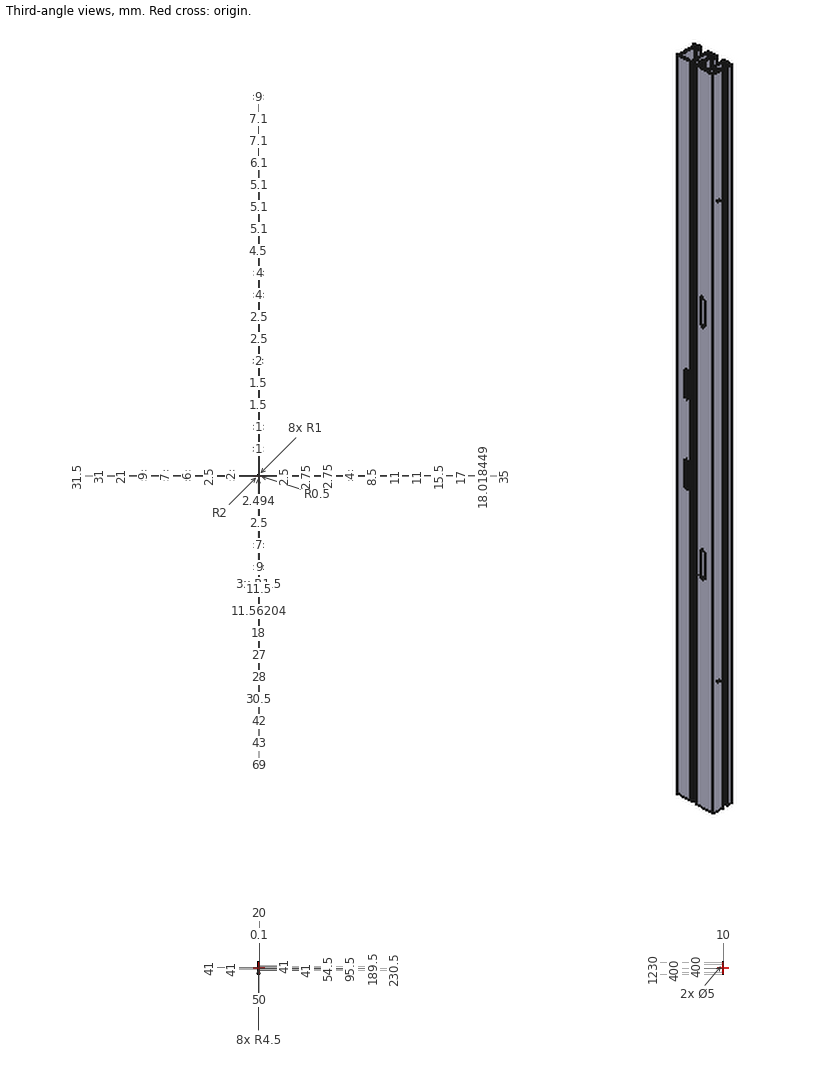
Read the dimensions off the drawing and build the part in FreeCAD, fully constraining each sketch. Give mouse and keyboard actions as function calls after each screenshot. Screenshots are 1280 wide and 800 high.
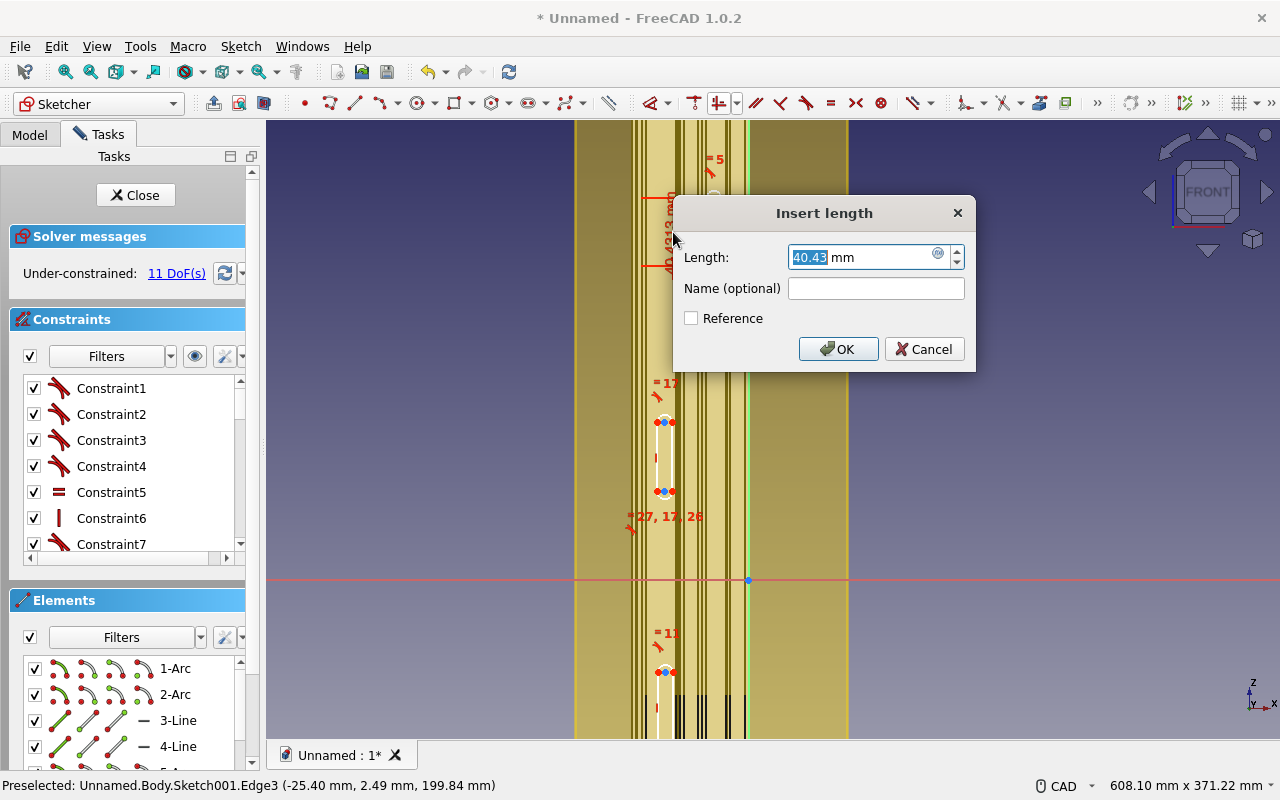
text(41)
key(Return)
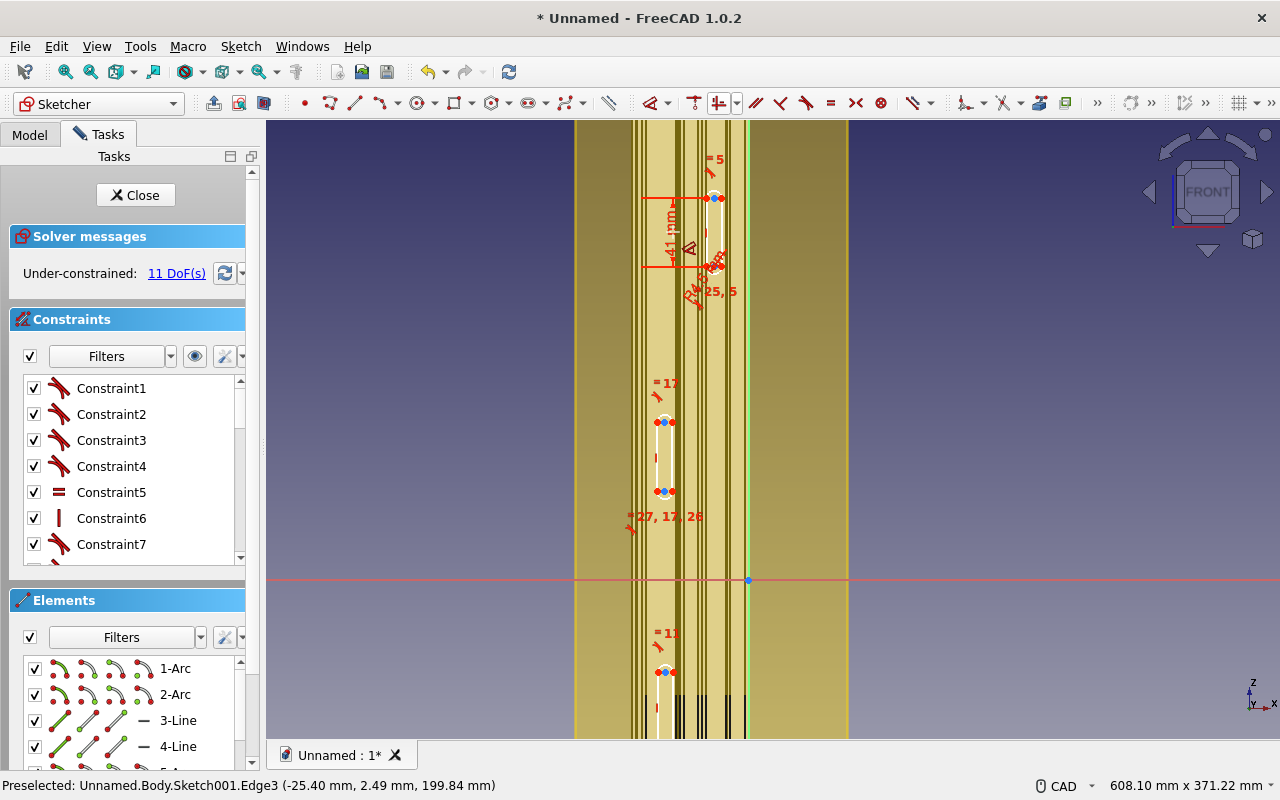
click(658, 693)
click(624, 692)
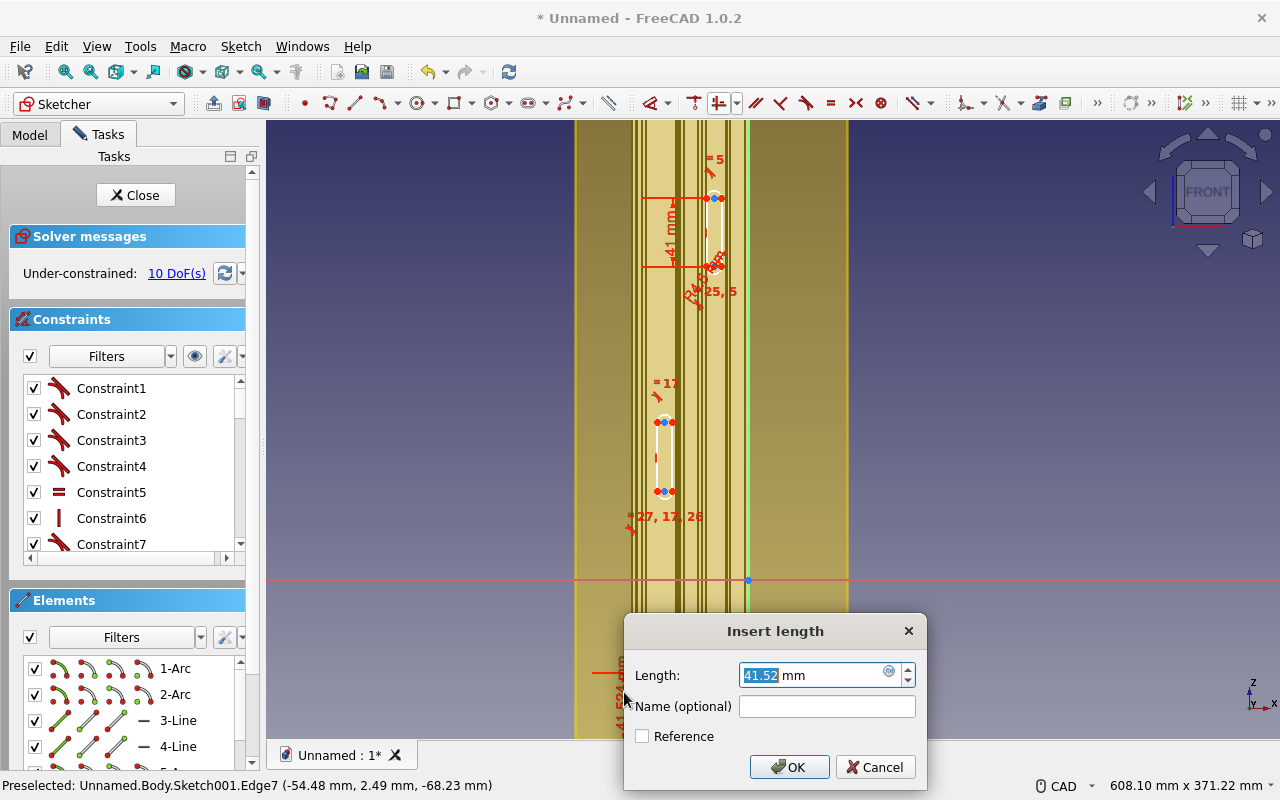
text(41)
key(Return)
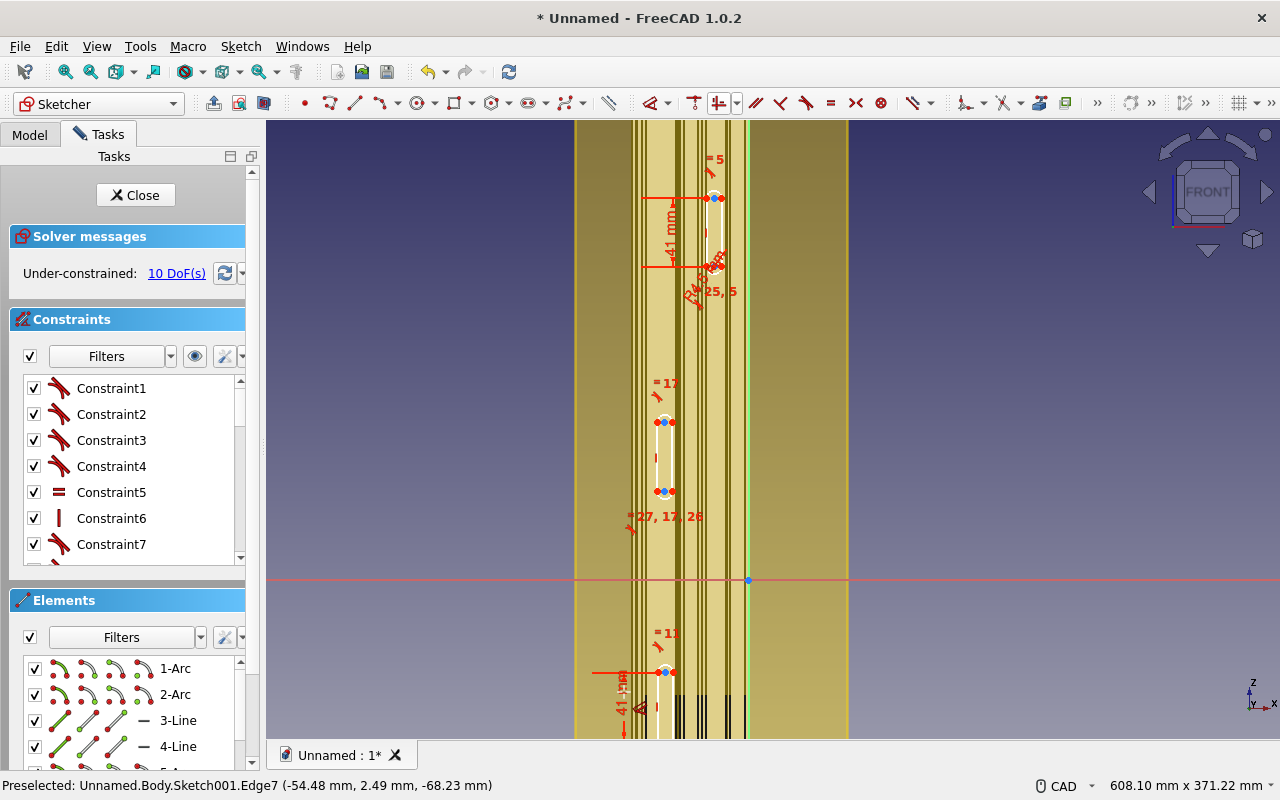
click(657, 471)
click(623, 457)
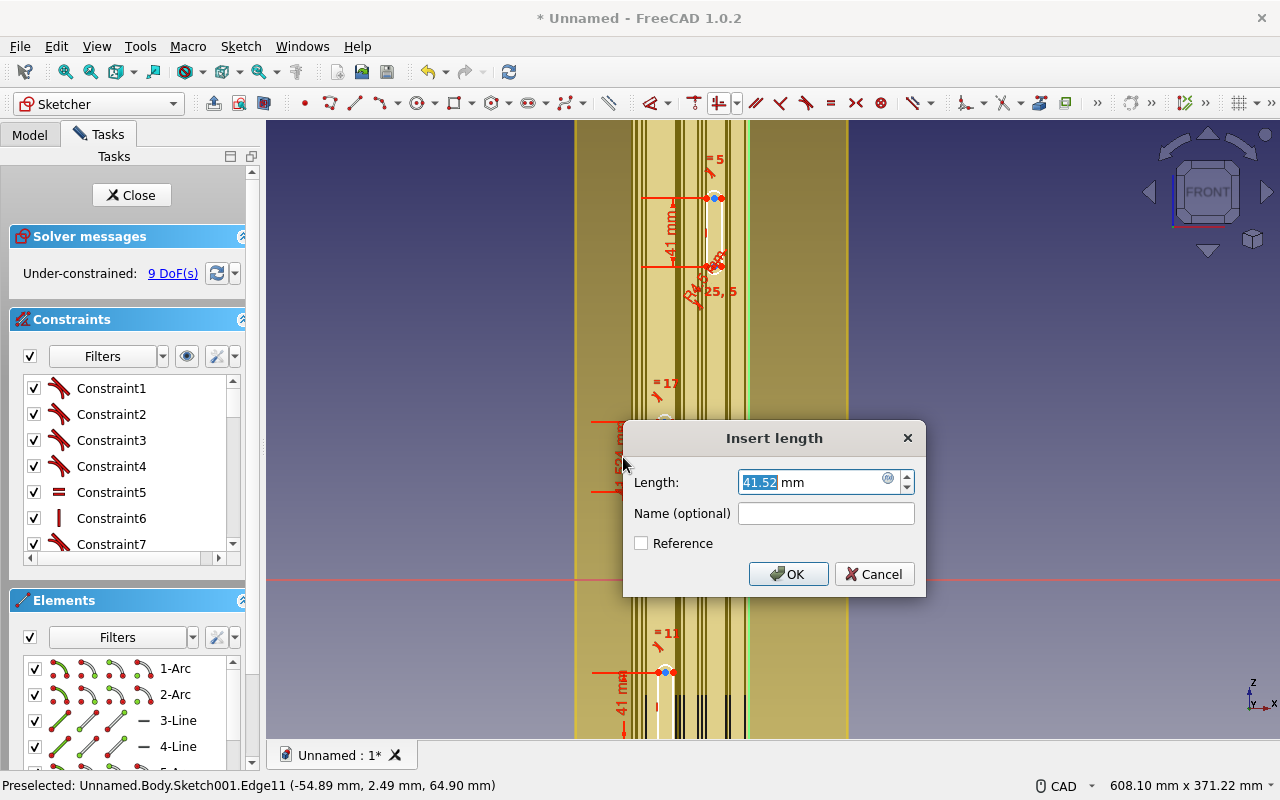
text(41)
key(Return)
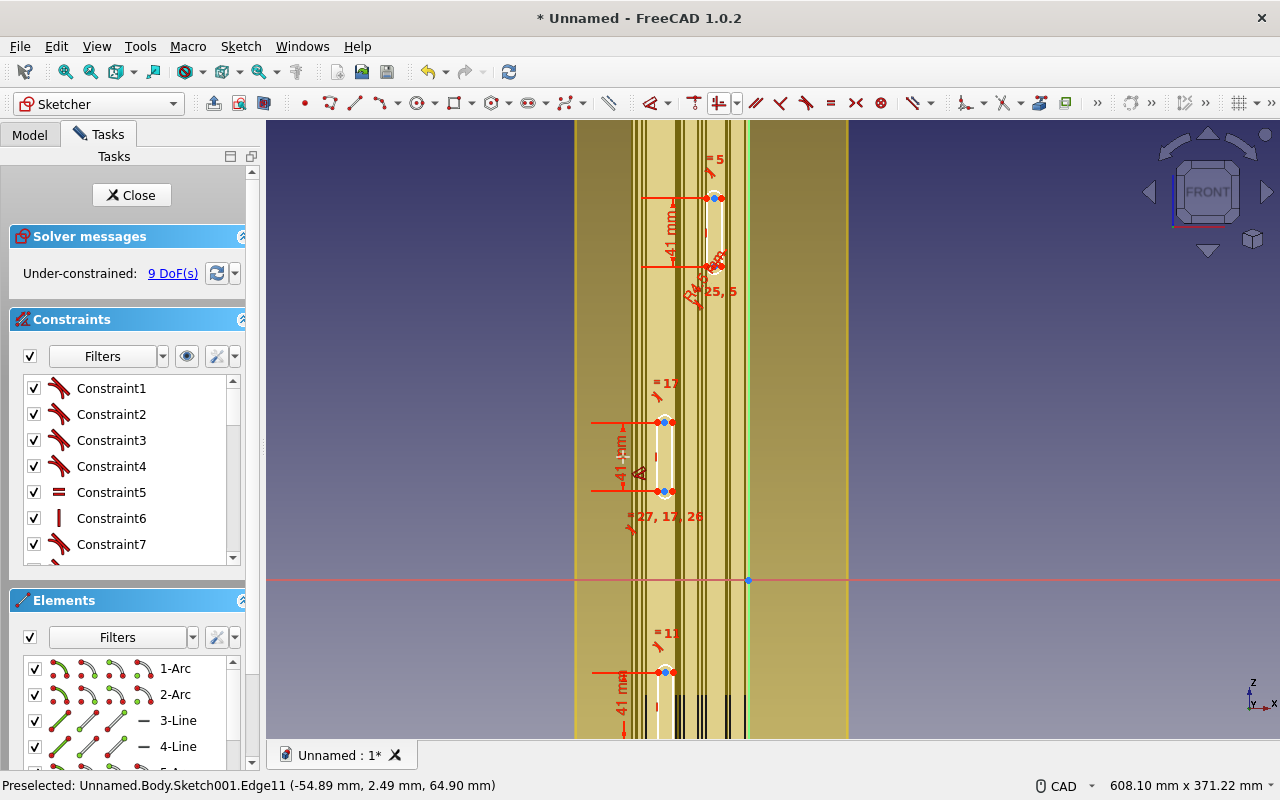
scroll(706, 246, down, 3)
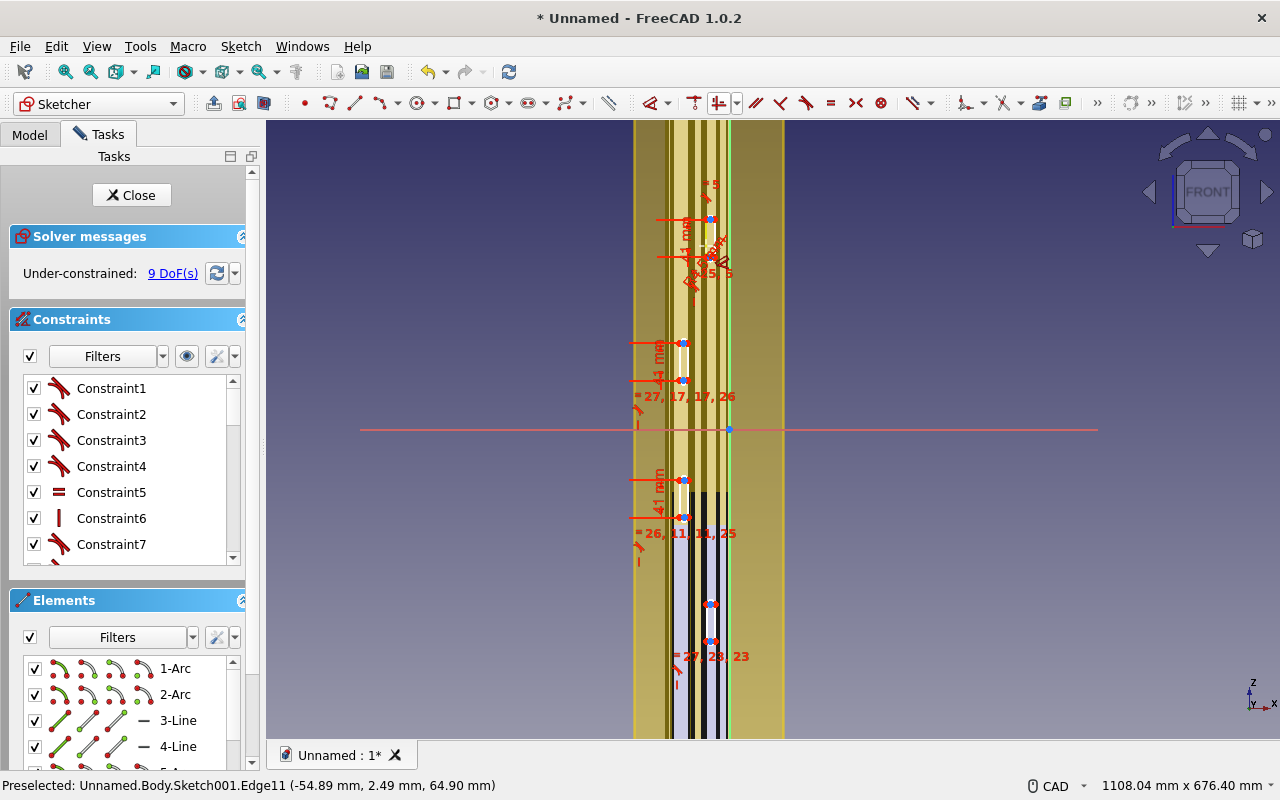
scroll(707, 630, up, 3)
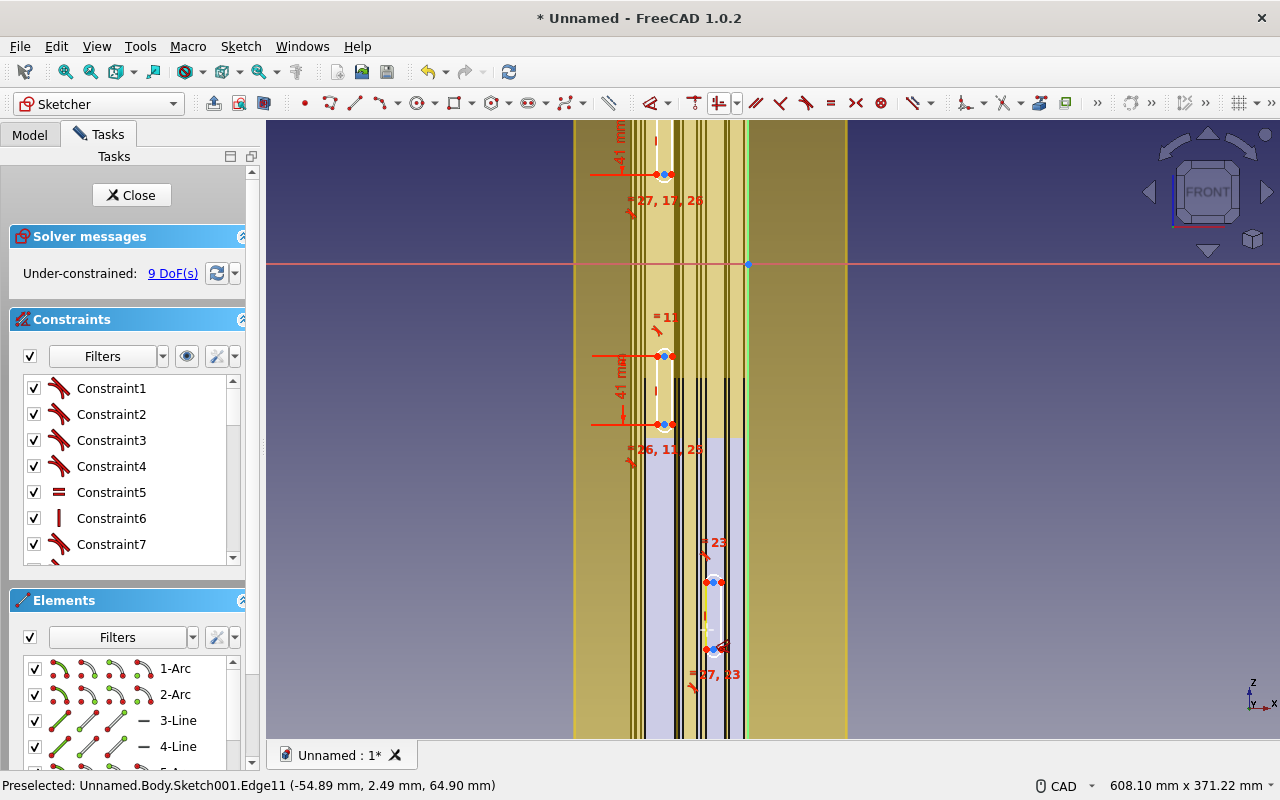
click(706, 629)
click(672, 616)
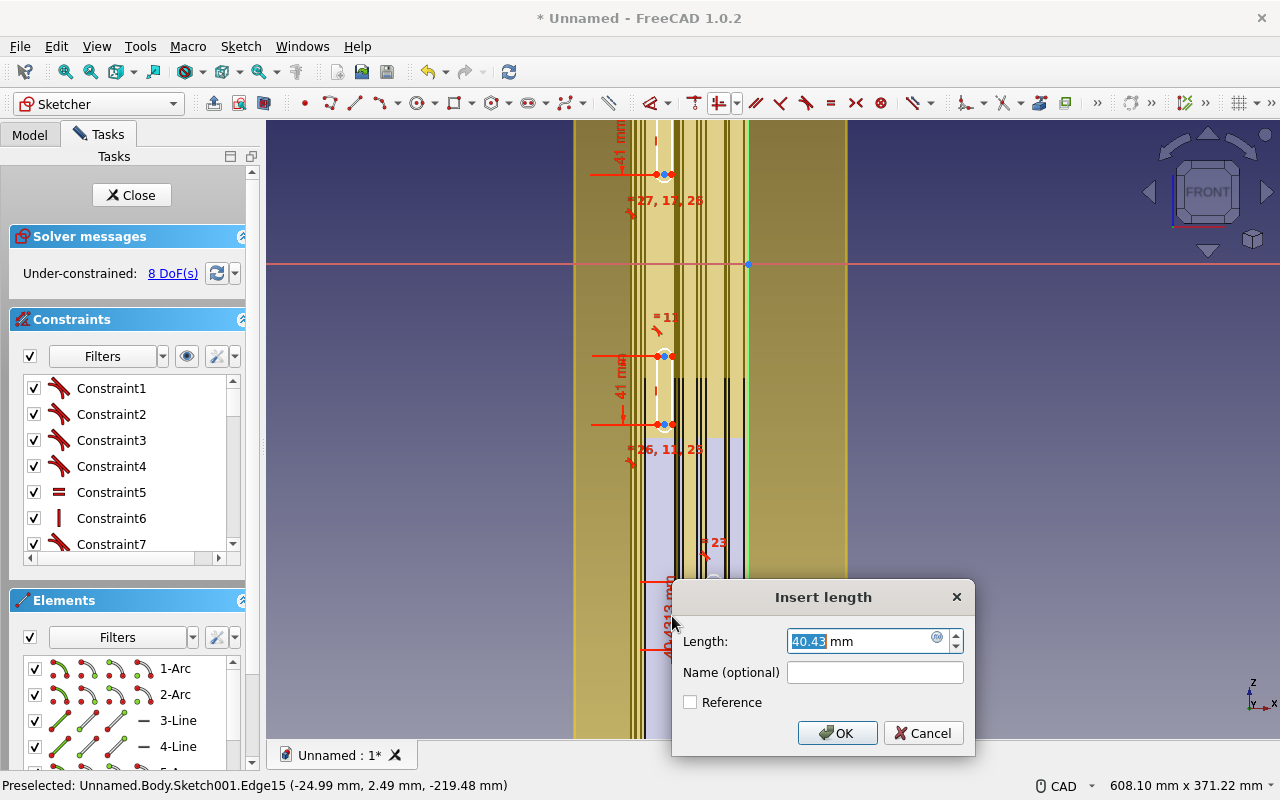
text(41)
key(Return)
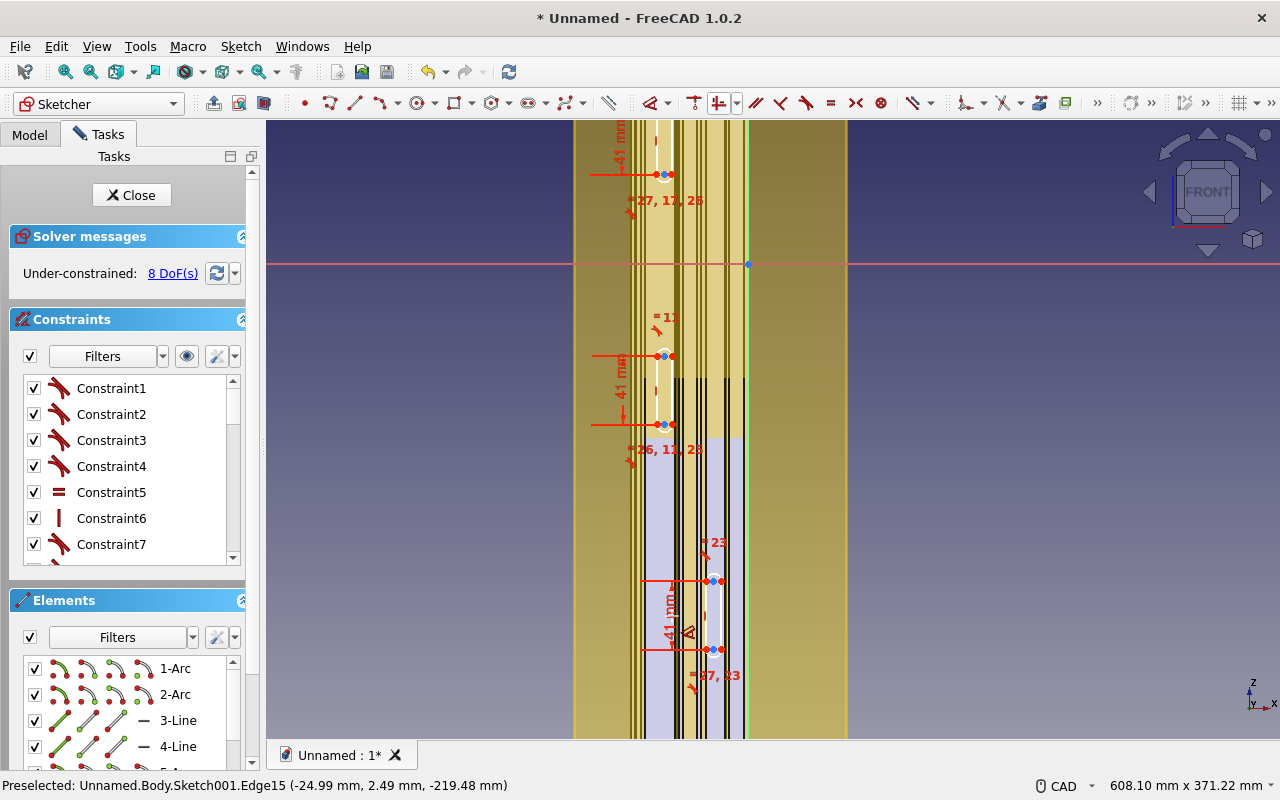
scroll(707, 631, down, 3)